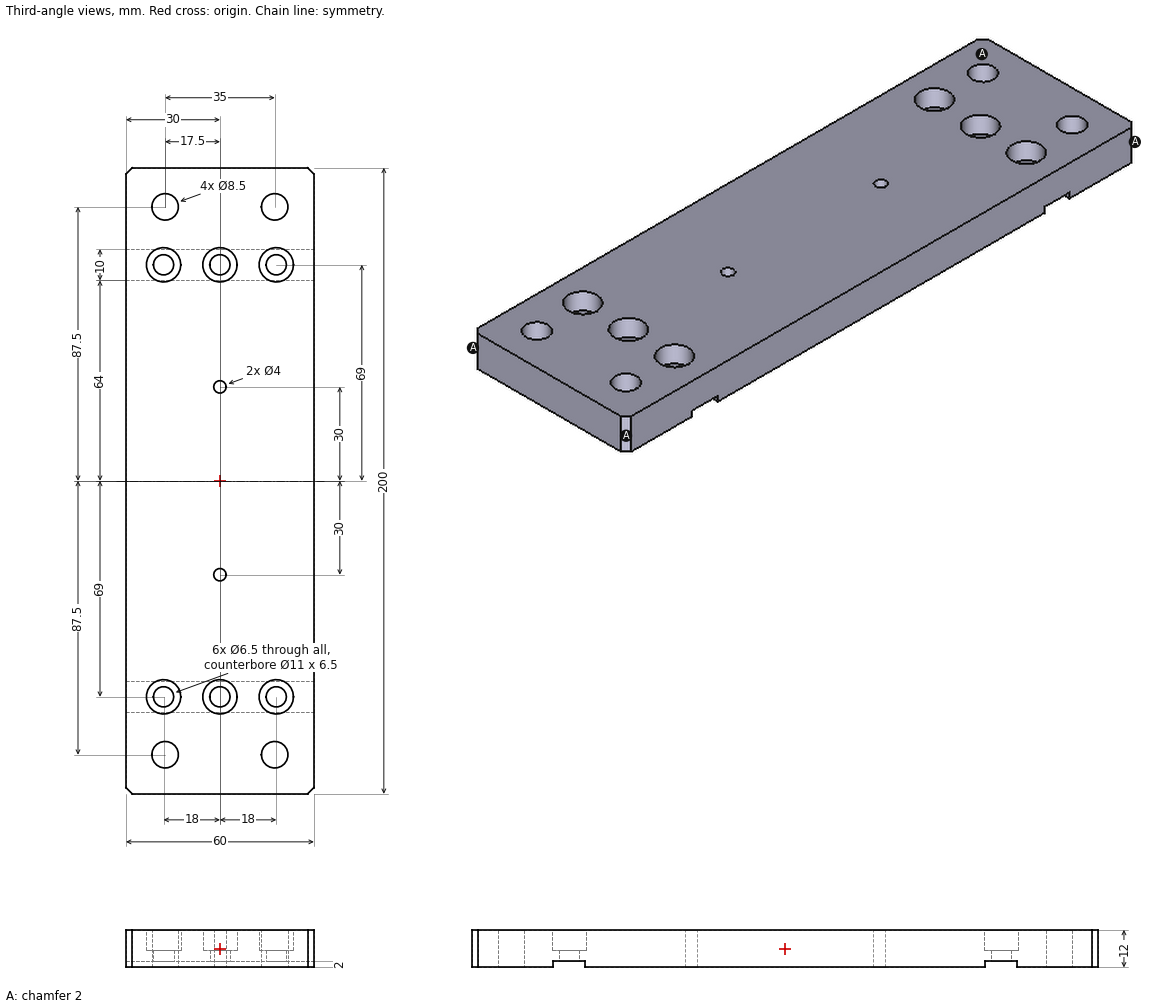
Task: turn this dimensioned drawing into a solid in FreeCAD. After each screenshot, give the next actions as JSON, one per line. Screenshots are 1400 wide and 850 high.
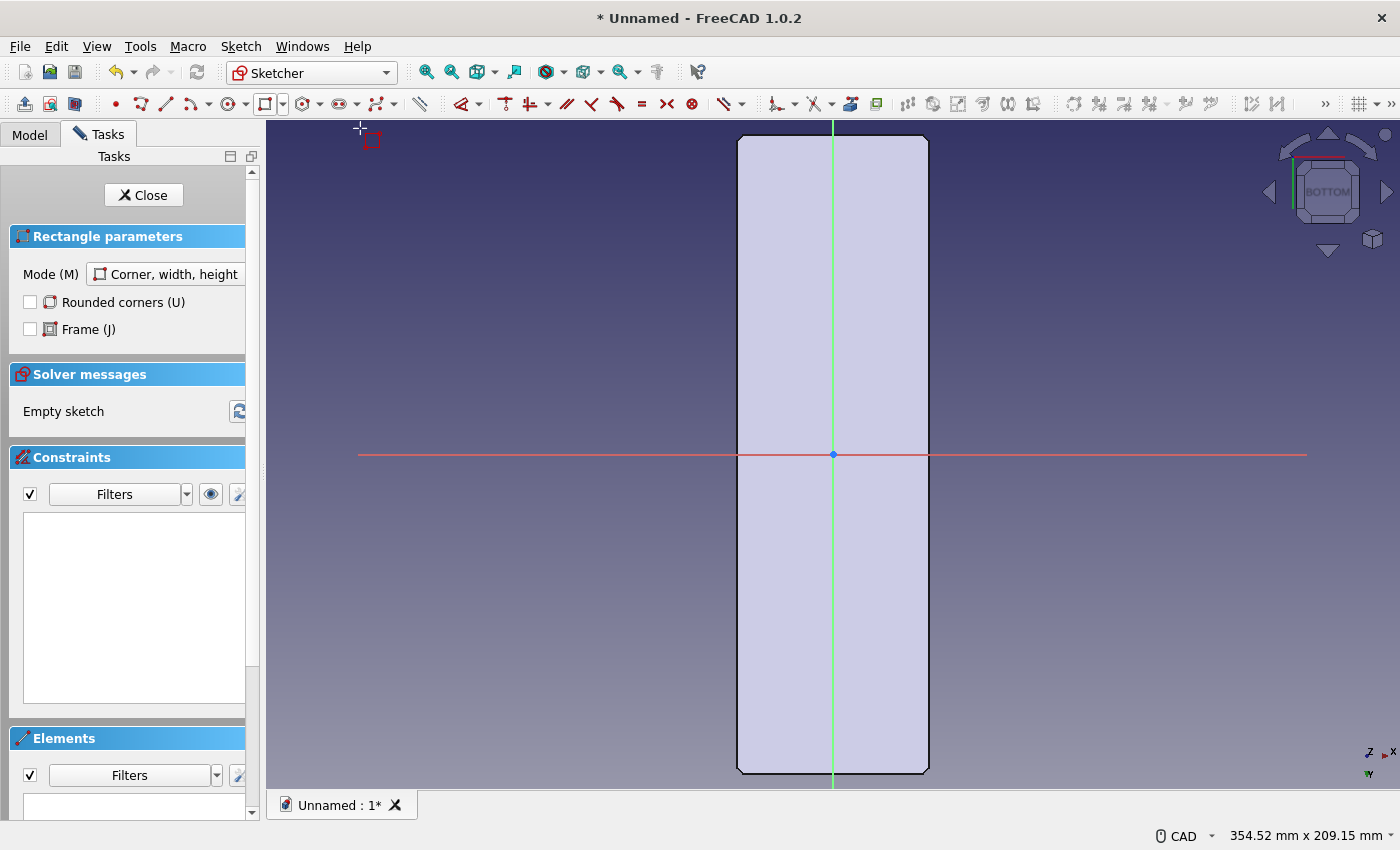
{"action": "left_click", "coordinate": [737, 659]}
{"action": "left_click", "coordinate": [929, 691]}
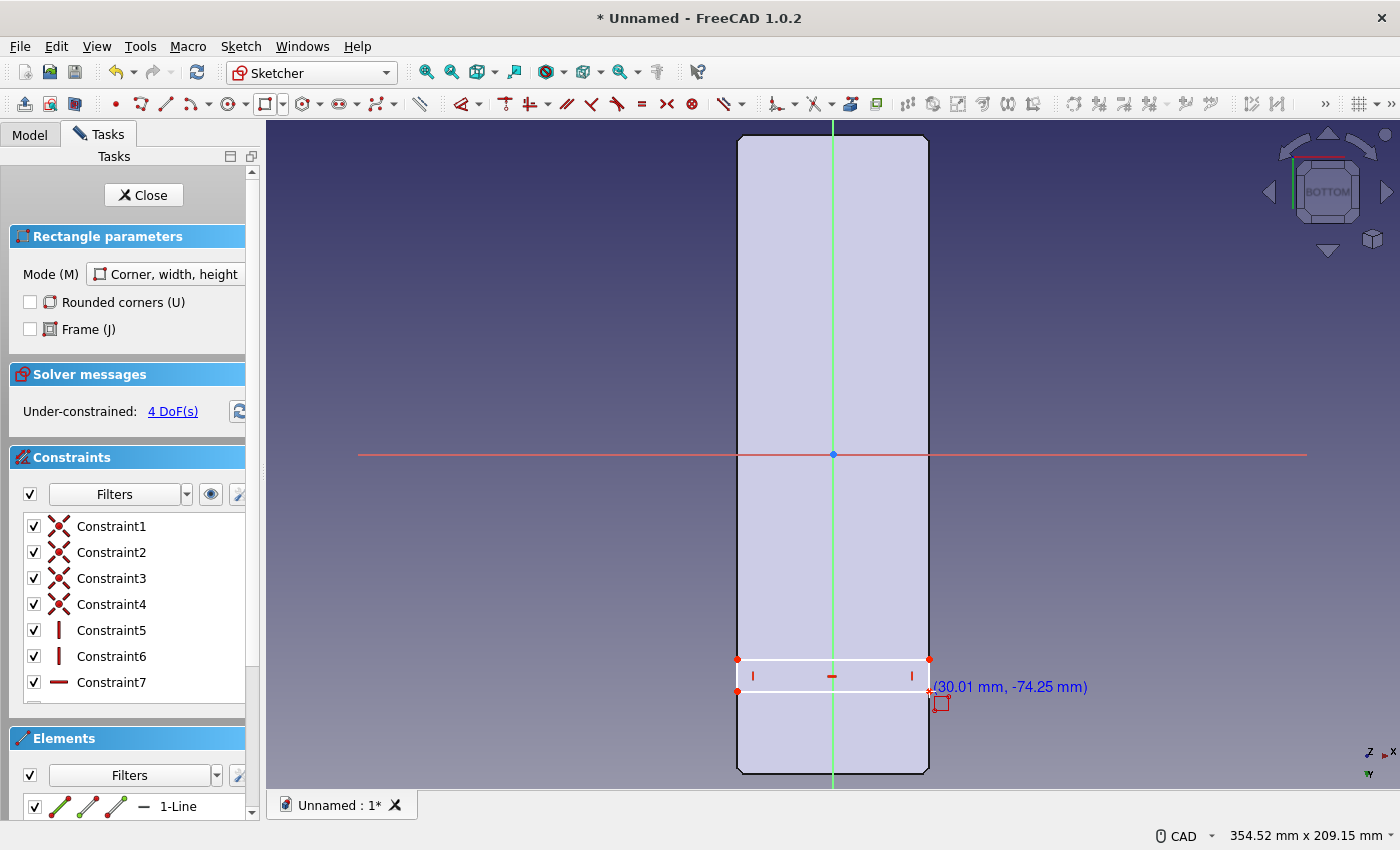
{"action": "left_click", "coordinate": [737, 218]}
{"action": "left_click", "coordinate": [929, 250]}
{"action": "key", "text": "Escape"}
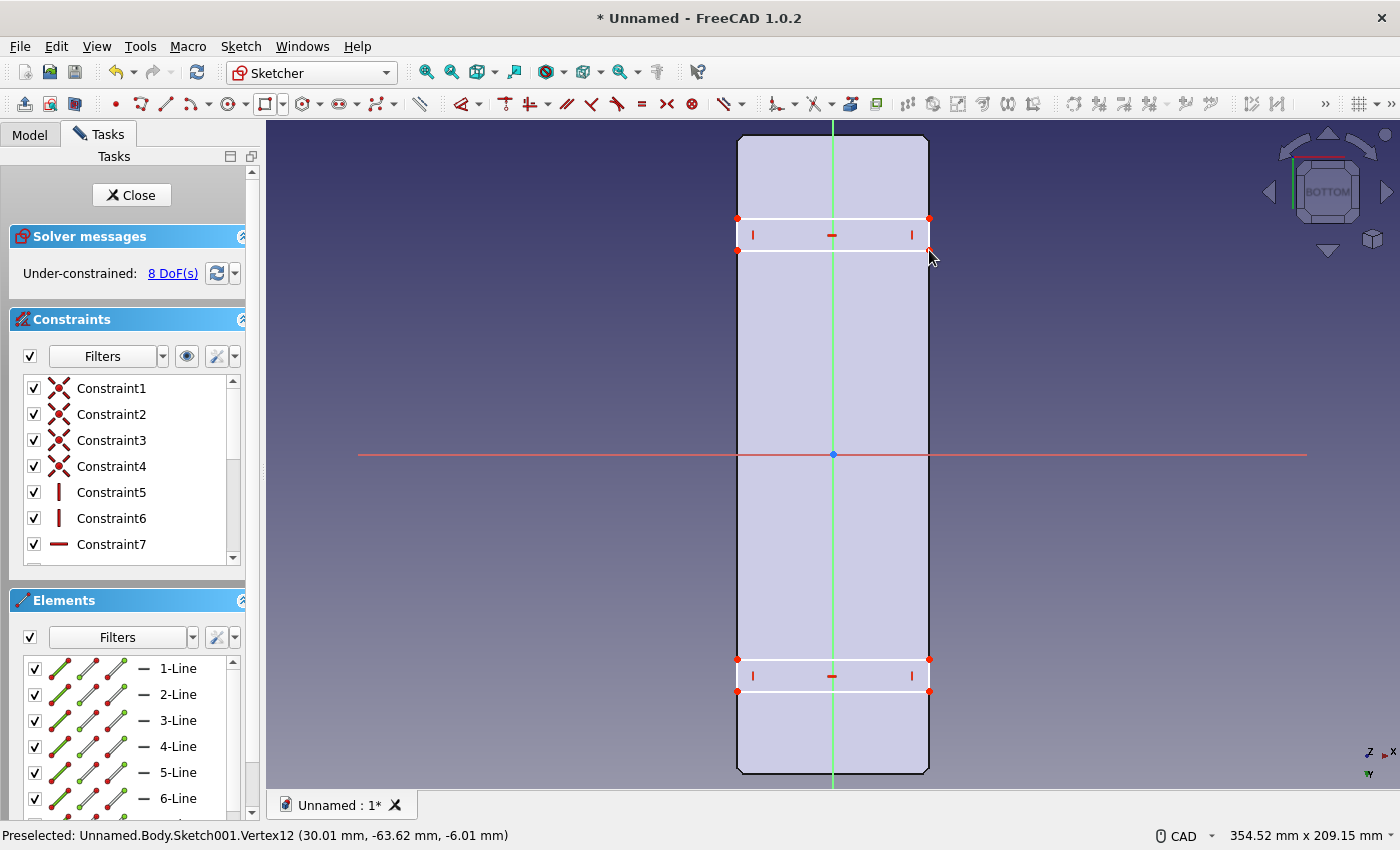
{"action": "left_click", "coordinate": [737, 692]}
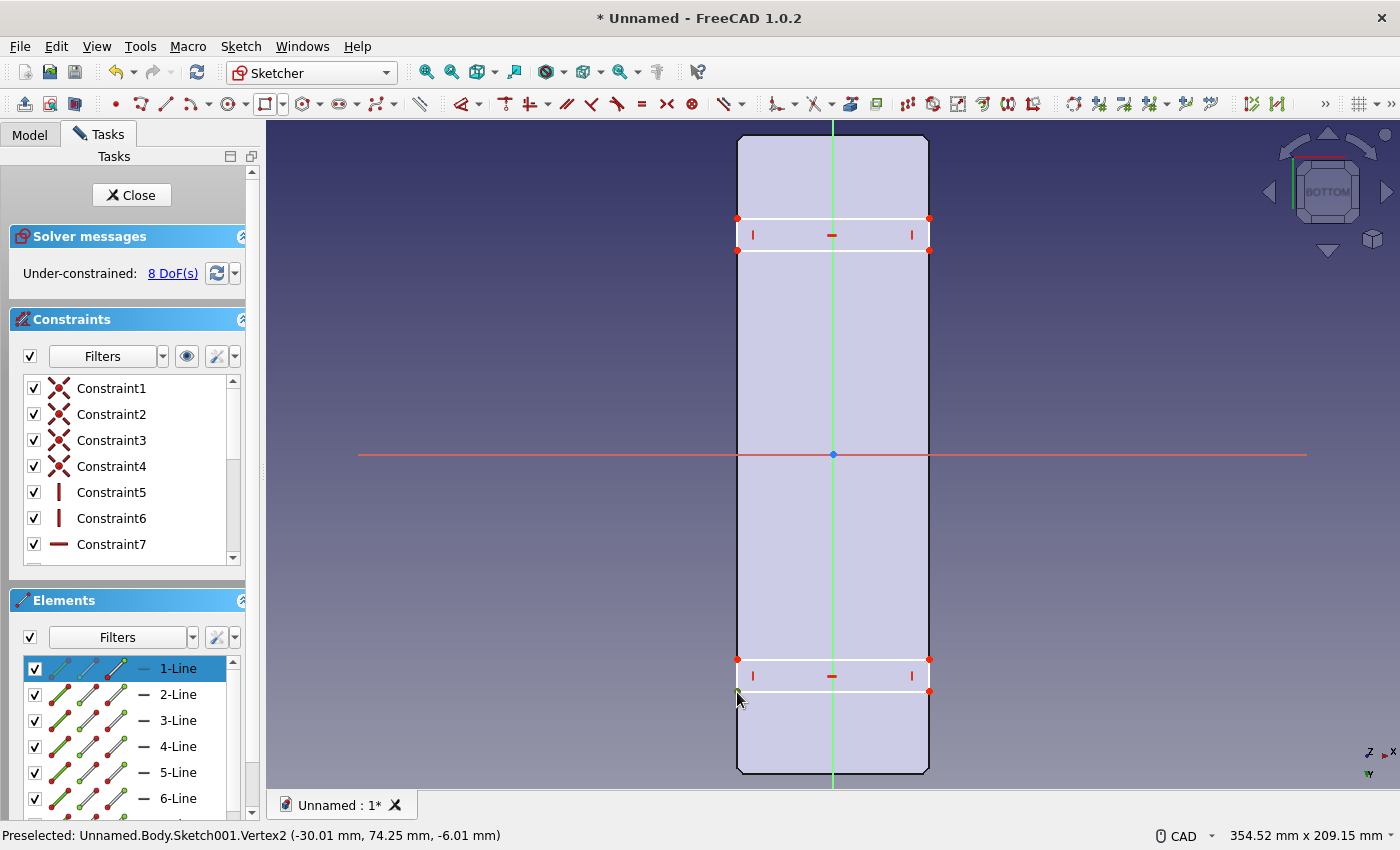
{"action": "left_click", "coordinate": [737, 219]}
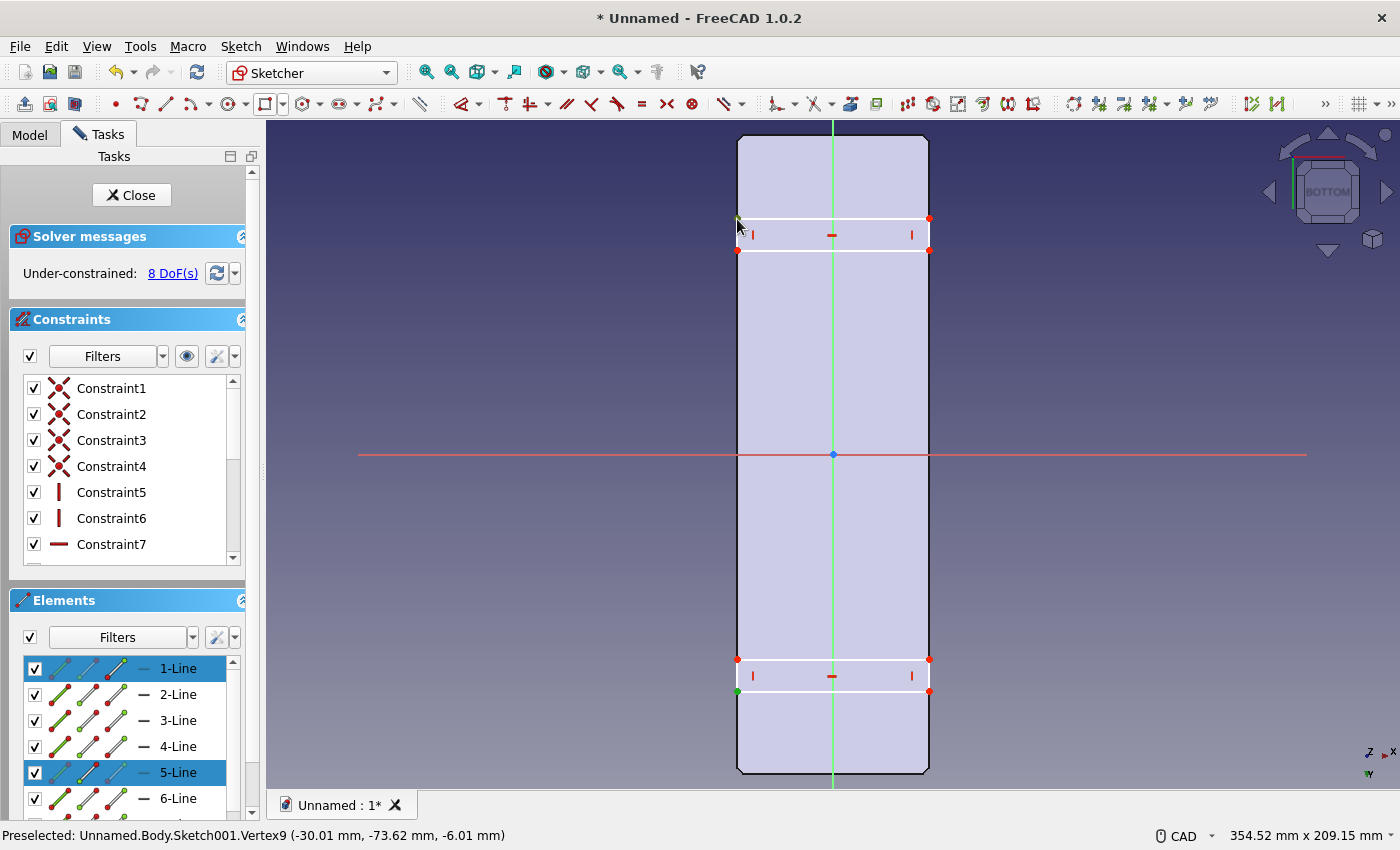
{"action": "left_click", "coordinate": [361, 454]}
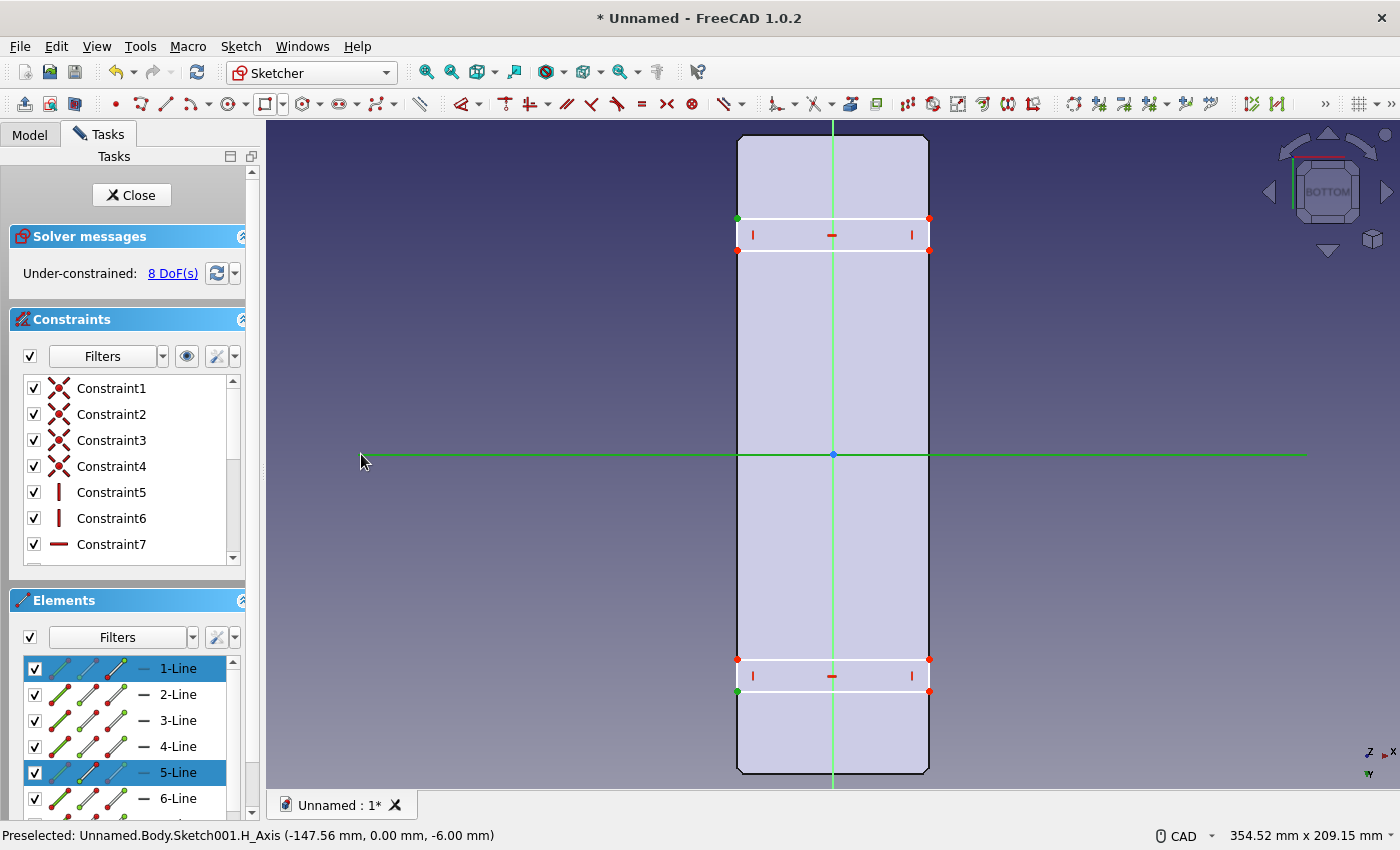
{"action": "left_click", "coordinate": [667, 104]}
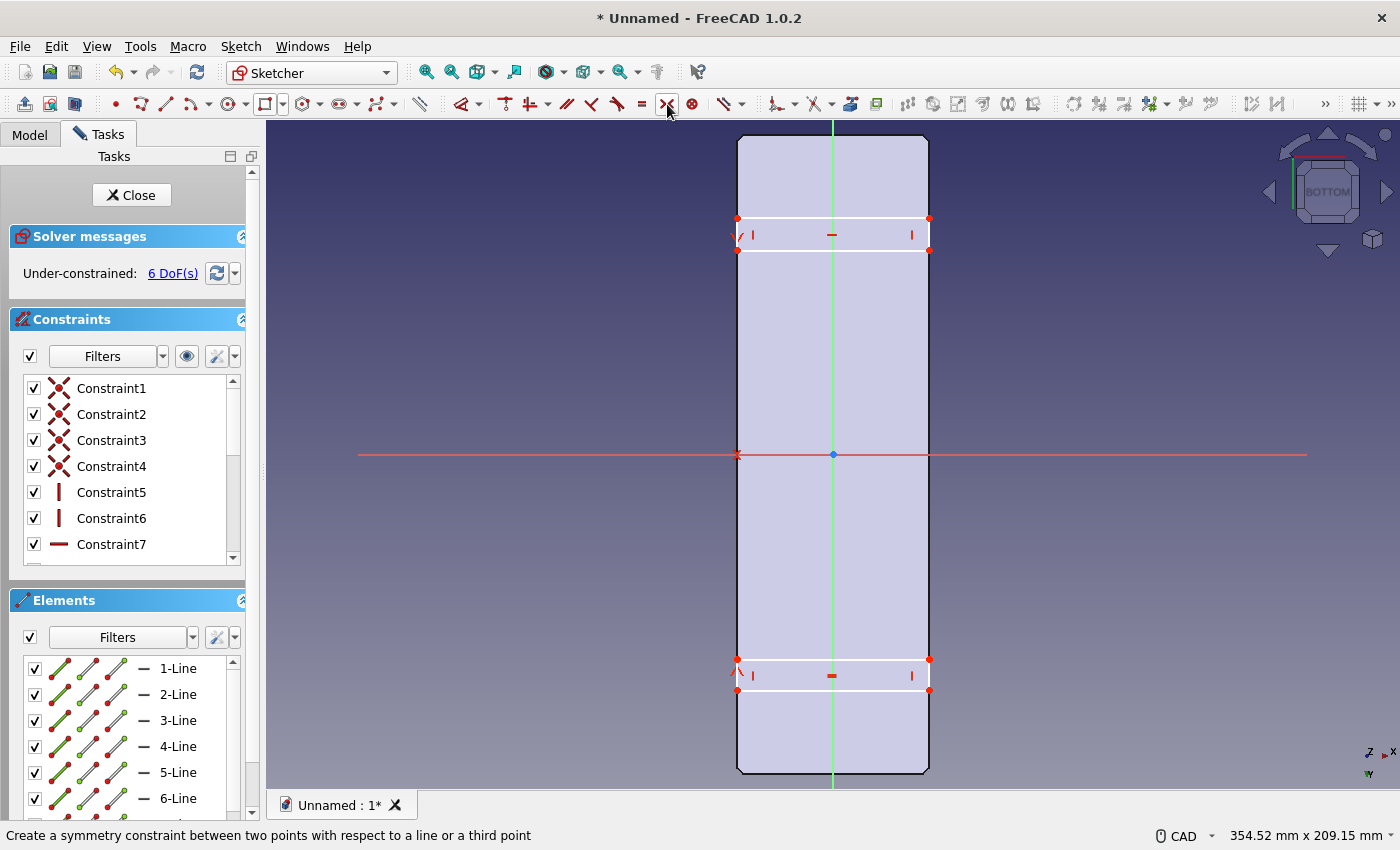
{"action": "left_click", "coordinate": [929, 660]}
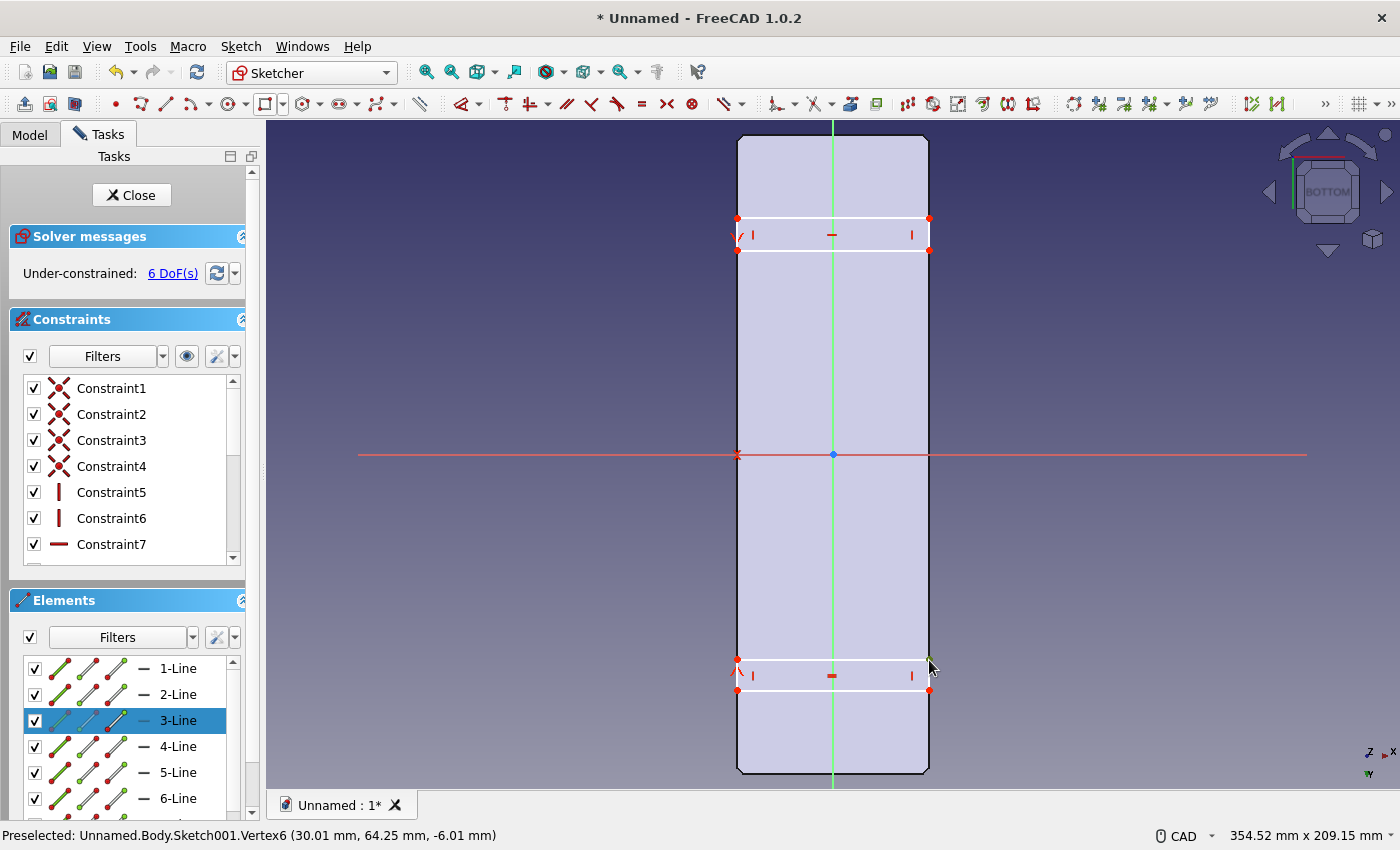
{"action": "left_click", "coordinate": [929, 251]}